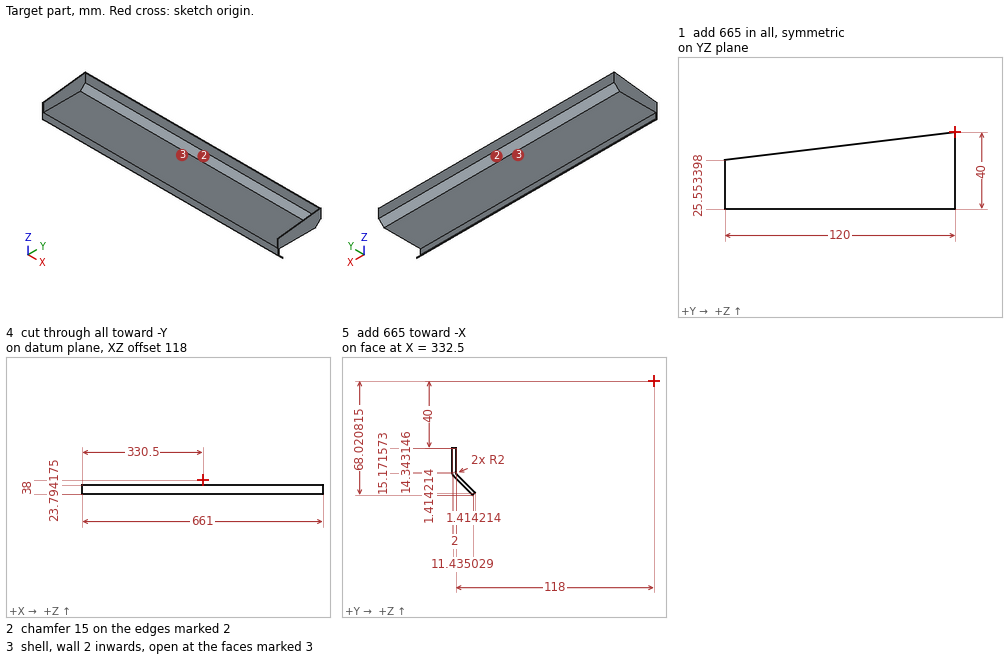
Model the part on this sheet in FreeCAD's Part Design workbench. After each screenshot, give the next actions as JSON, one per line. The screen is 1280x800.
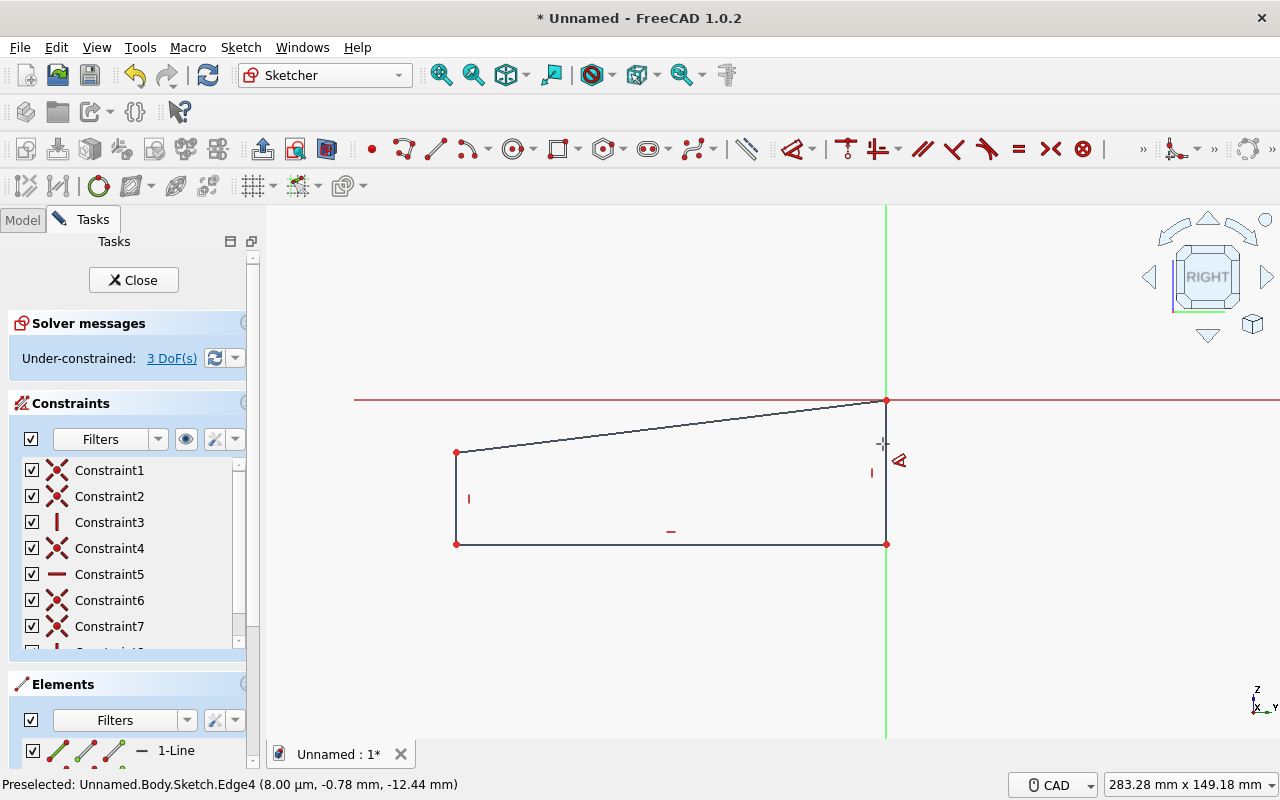
{"action": "left_click", "coordinate": [886, 502]}
{"action": "left_click", "coordinate": [920, 473]}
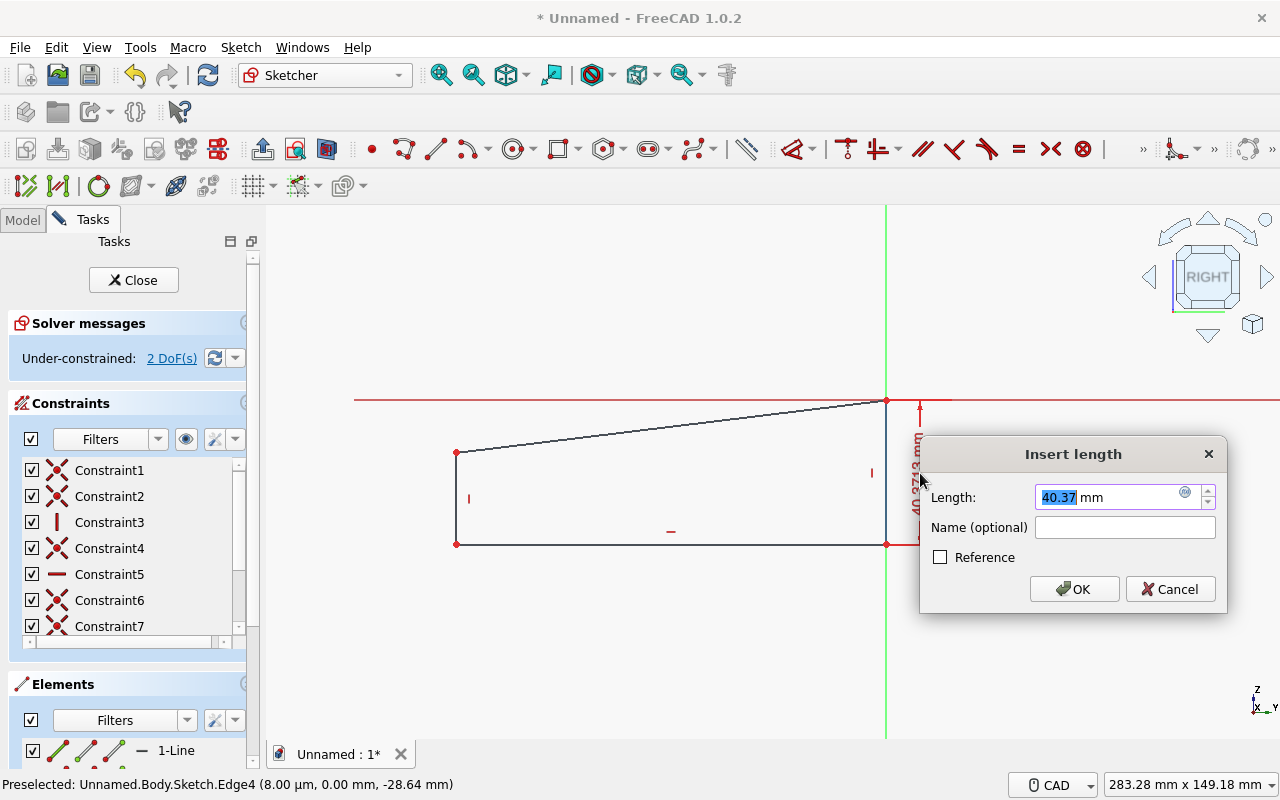
{"action": "type", "text": "40"}
{"action": "key", "text": "Return"}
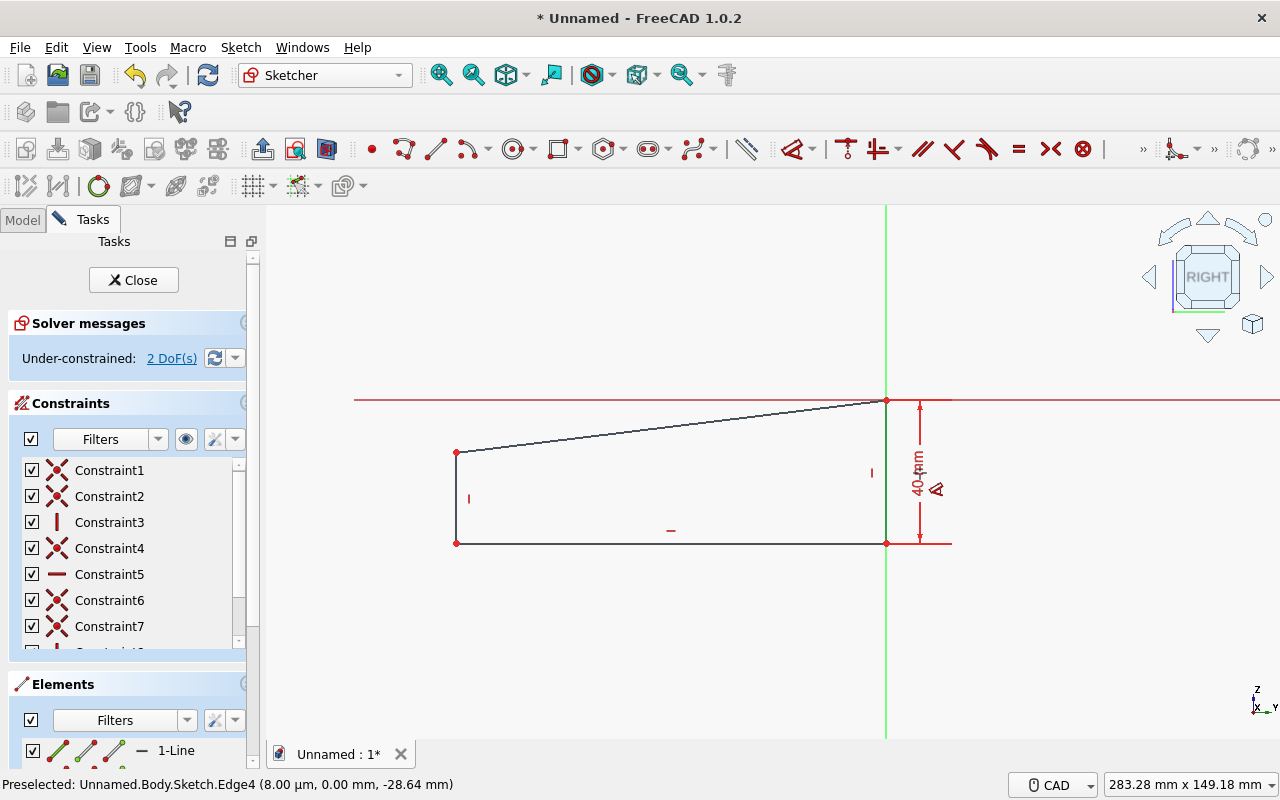
{"action": "left_click", "coordinate": [585, 544]}
{"action": "left_click", "coordinate": [671, 578]}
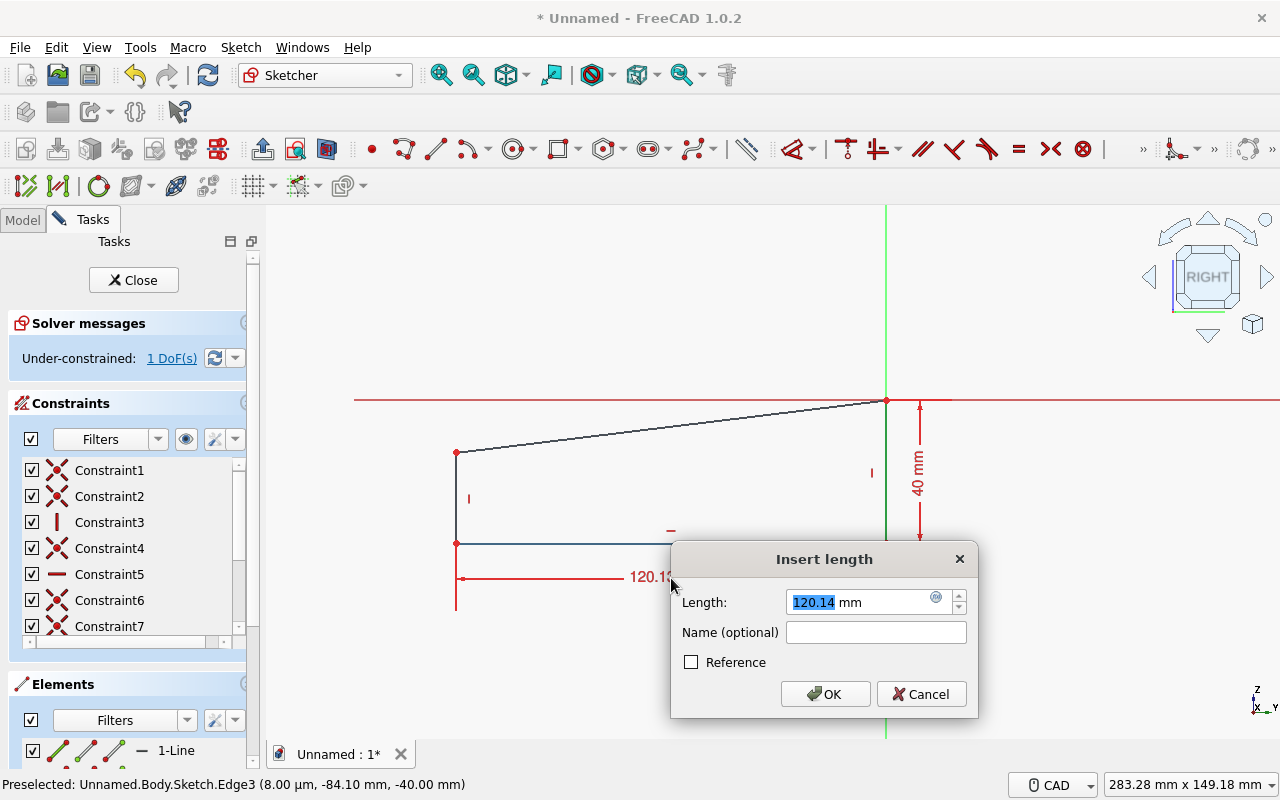
{"action": "type", "text": "120"}
{"action": "key", "text": "Return"}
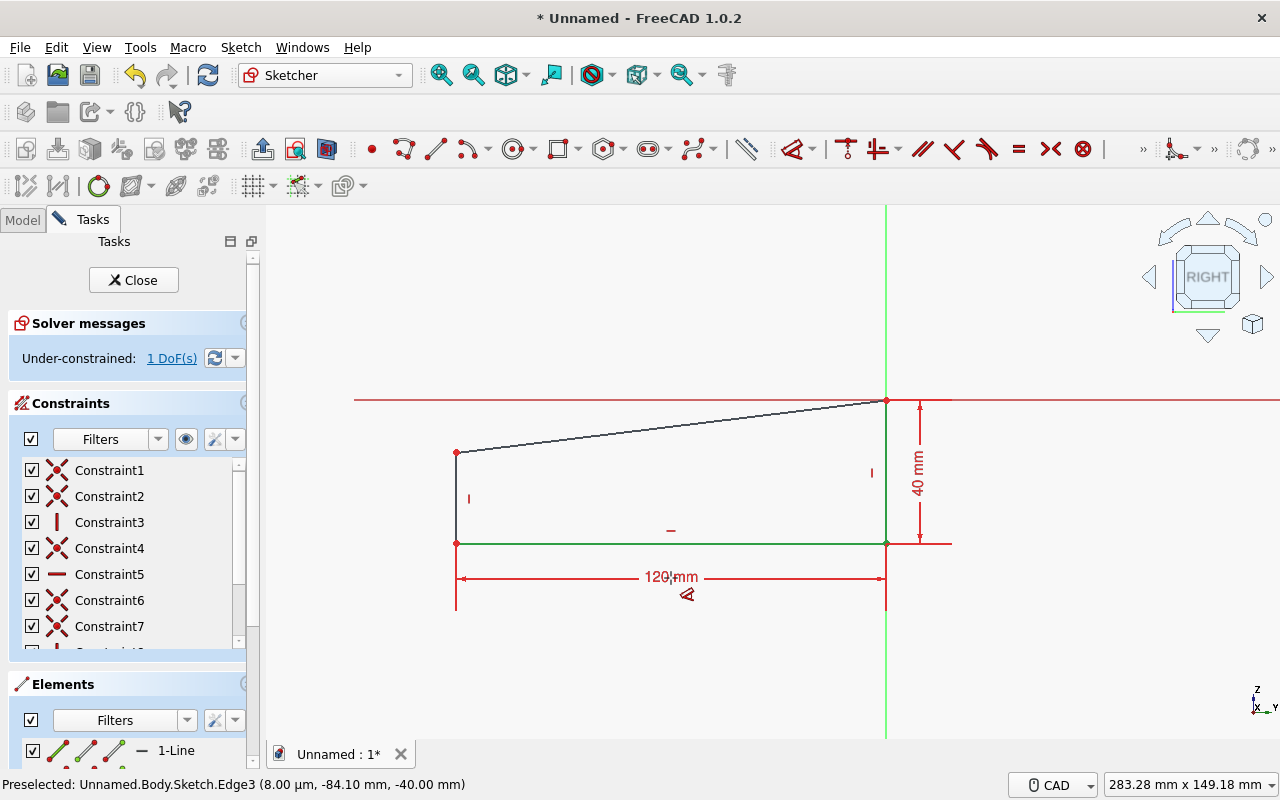
{"action": "left_click", "coordinate": [456, 480]}
{"action": "left_click", "coordinate": [422, 498]}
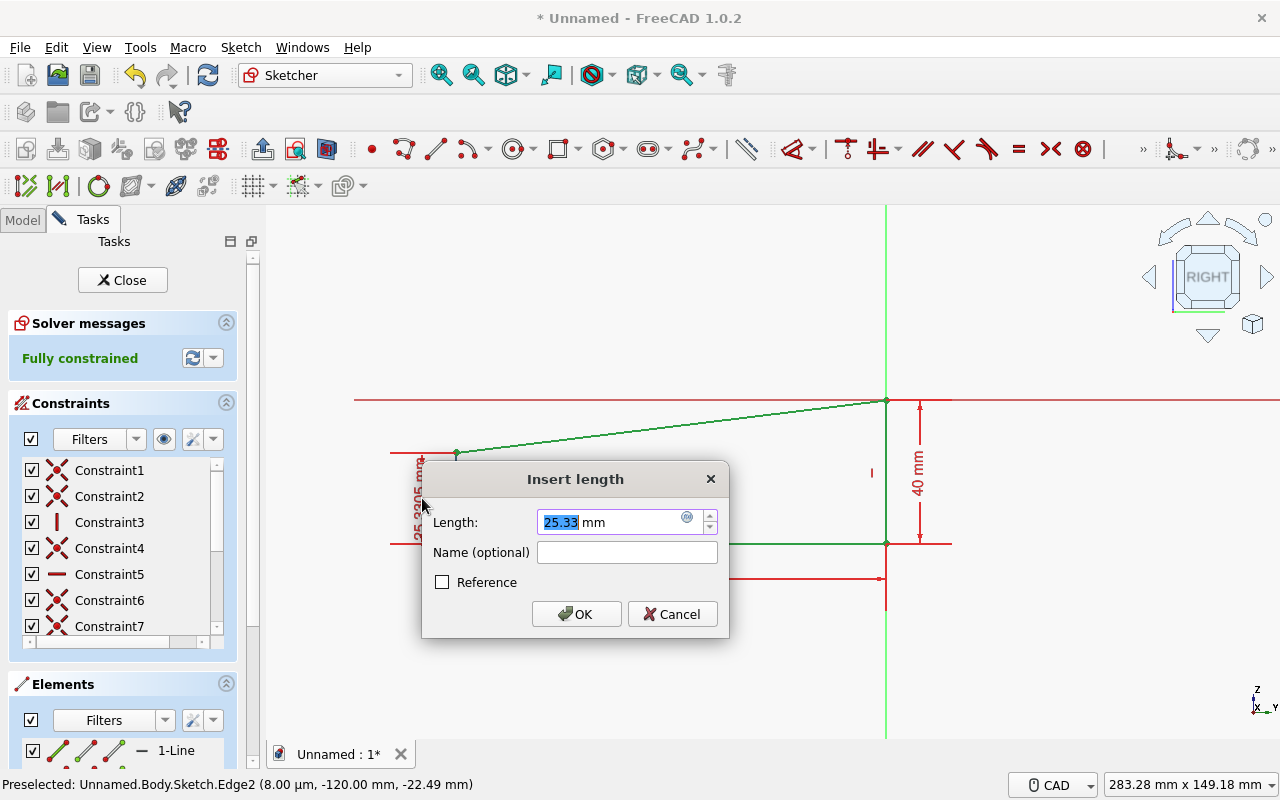
{"action": "type", "text": "25.553398"}
{"action": "key", "text": "Return"}
{"action": "key", "text": "Escape"}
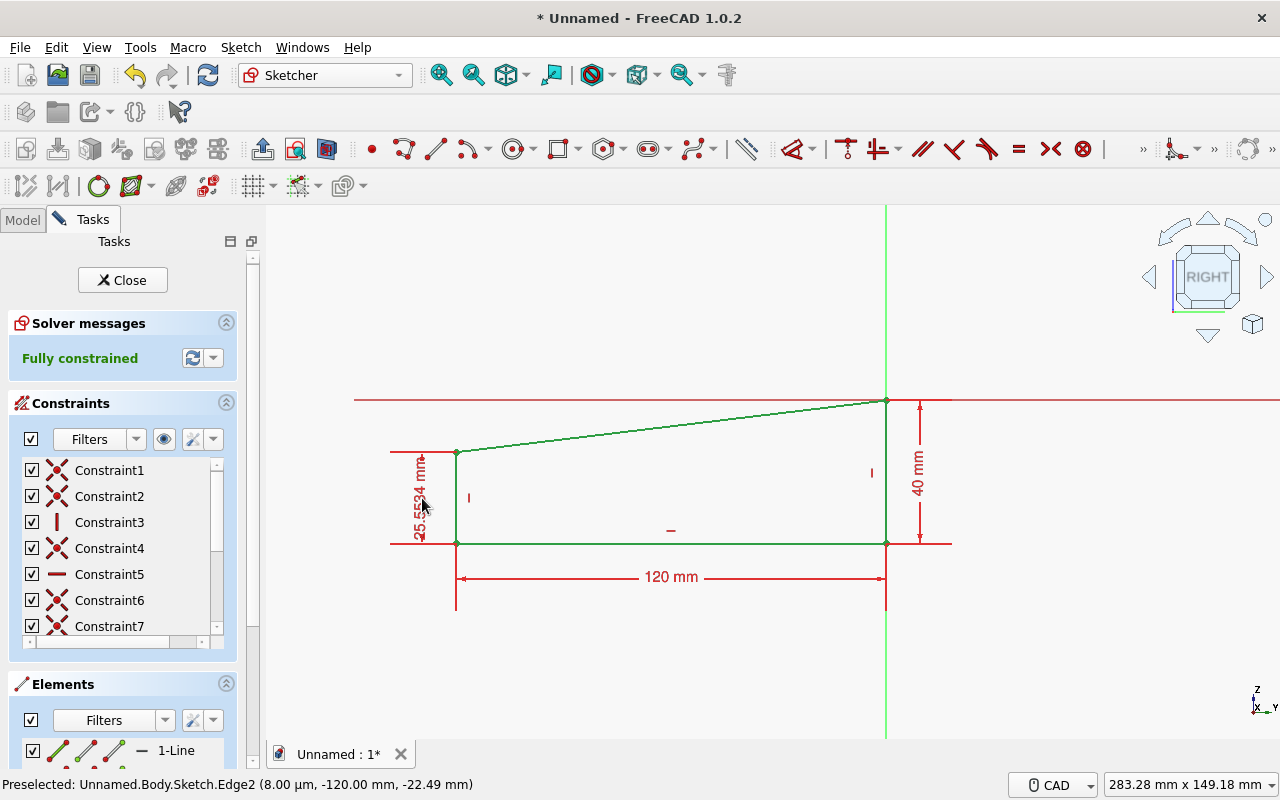
{"action": "left_click", "coordinate": [123, 280]}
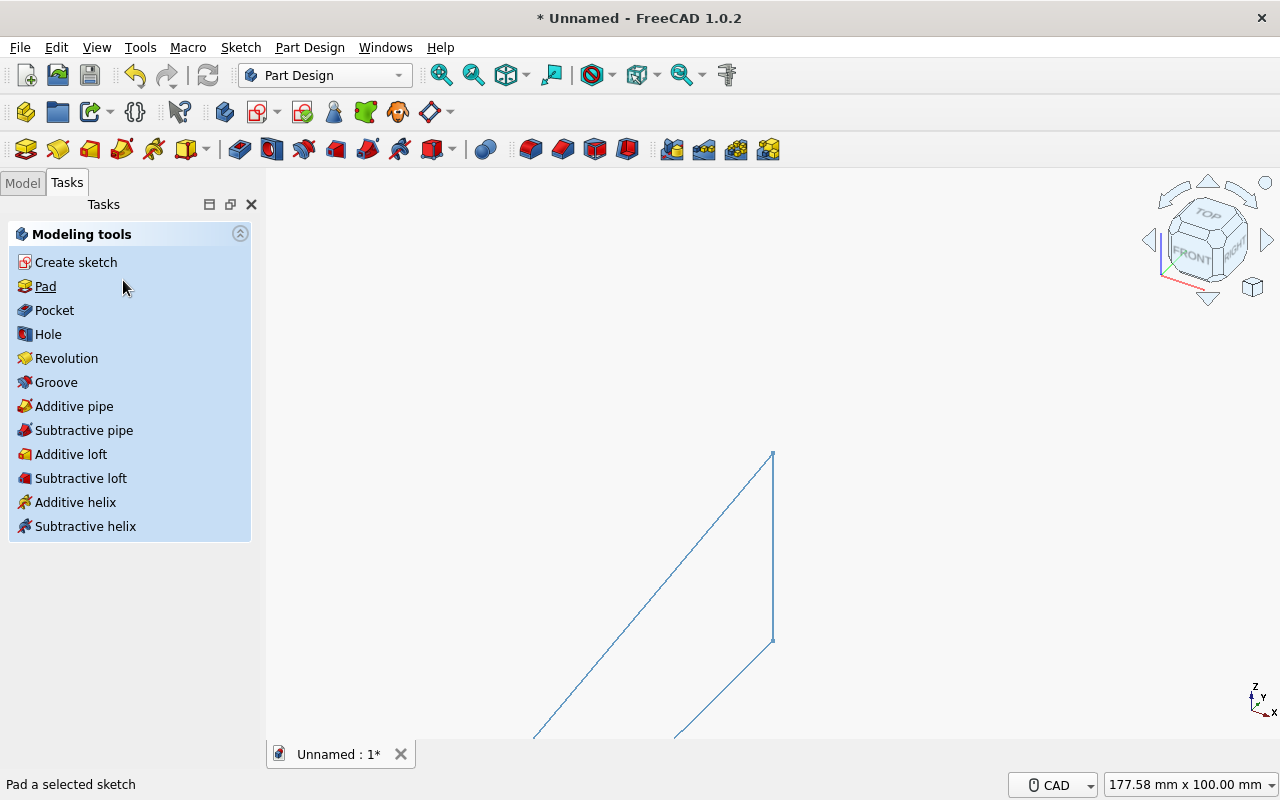
{"action": "left_click", "coordinate": [26, 150]}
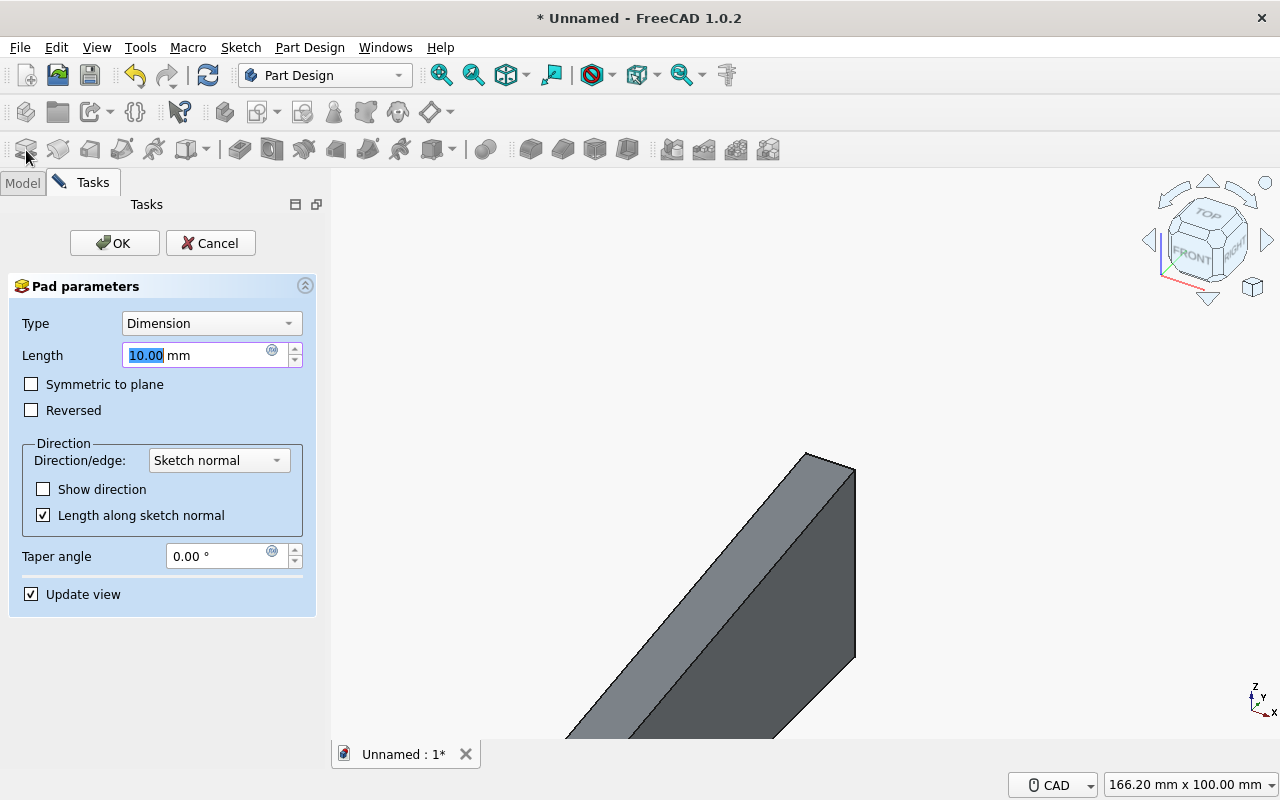
{"action": "type", "text": "665"}
{"action": "key", "text": "Tab"}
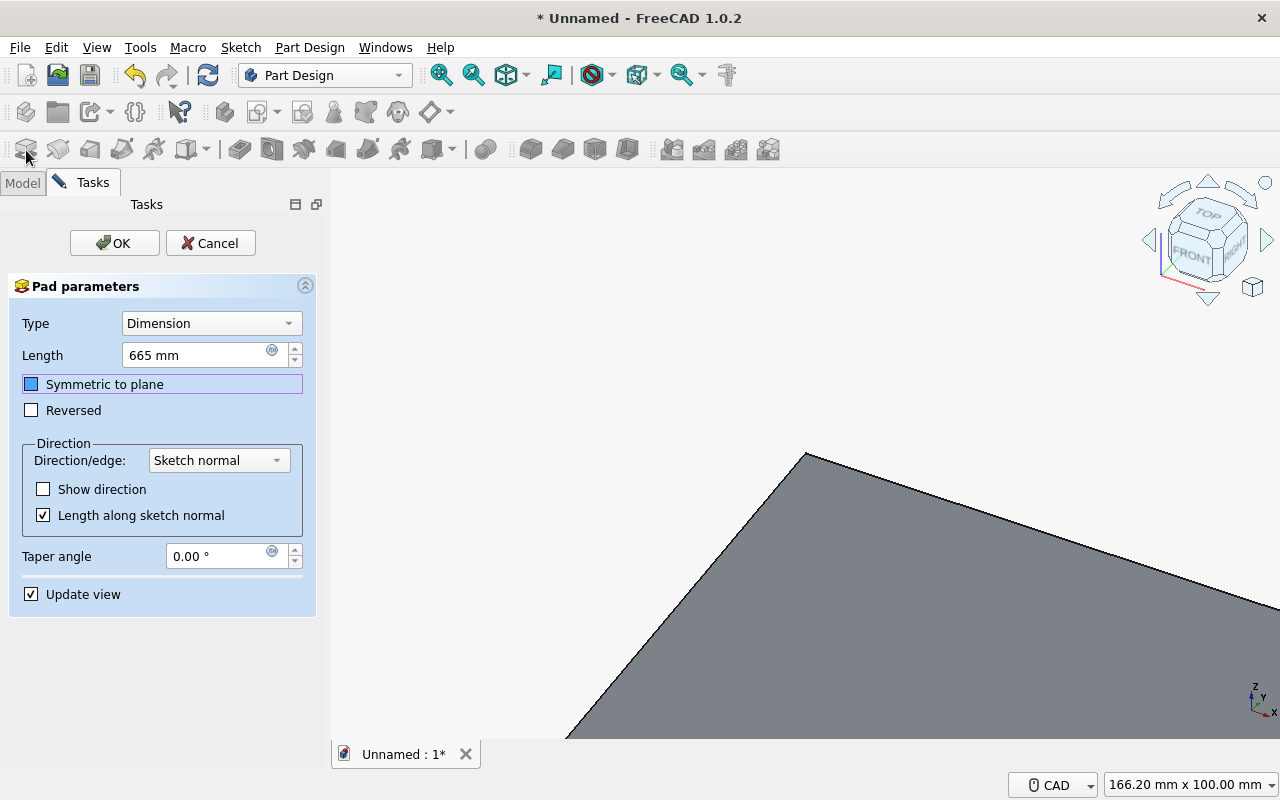
{"action": "left_click", "coordinate": [30, 384]}